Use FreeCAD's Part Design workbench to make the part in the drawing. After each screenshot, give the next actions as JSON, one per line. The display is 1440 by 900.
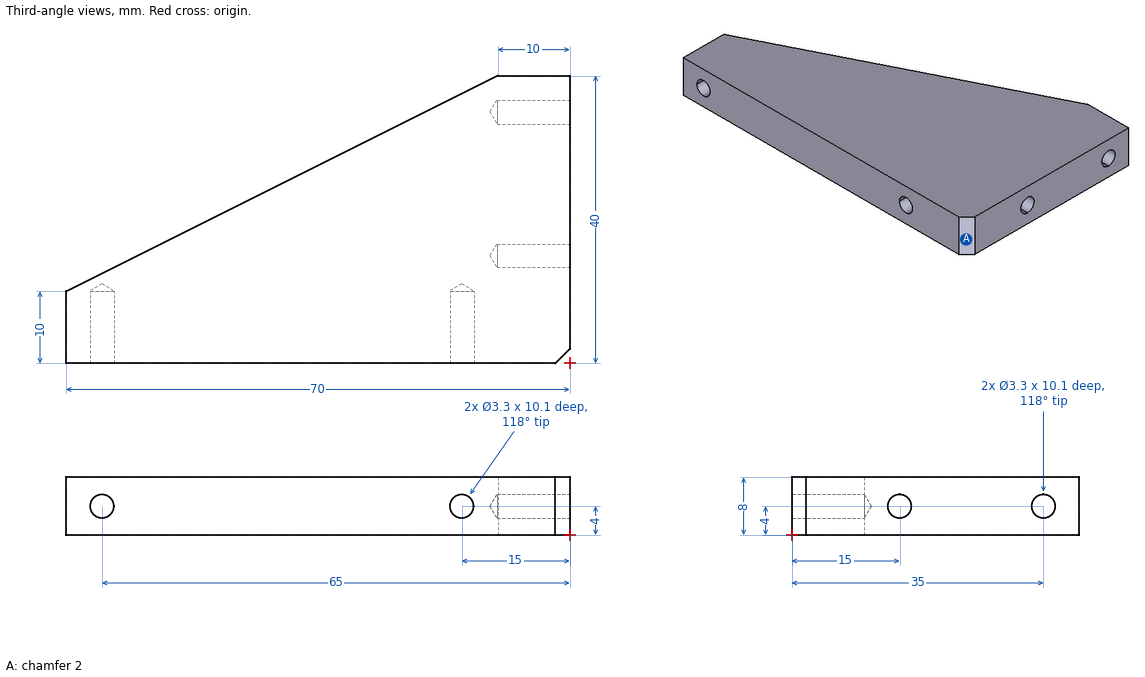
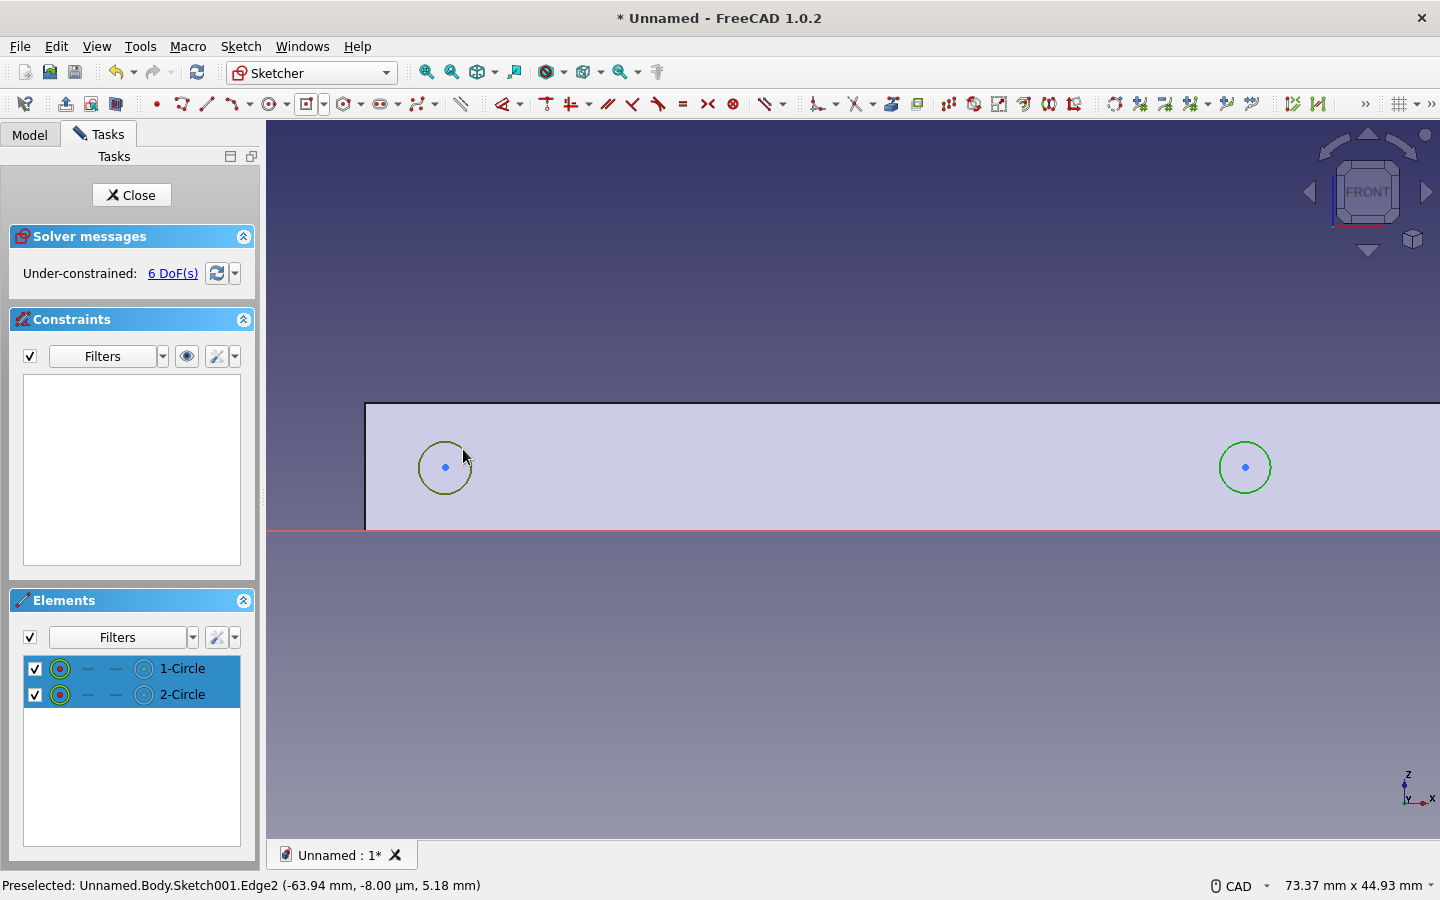
{"action": "left_click", "coordinate": [683, 104]}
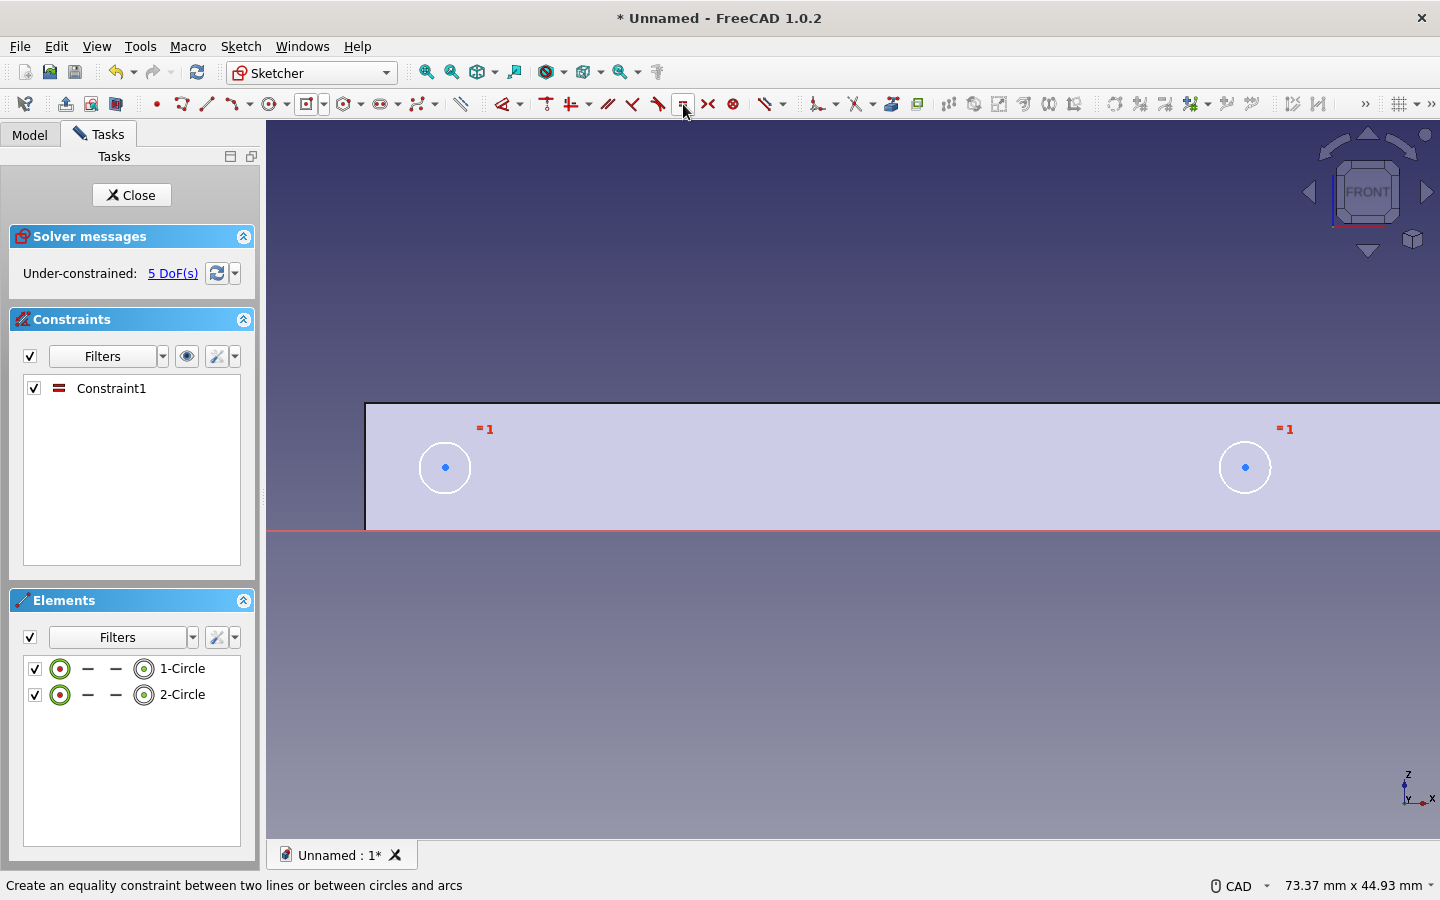
{"action": "left_click", "coordinate": [1245, 467]}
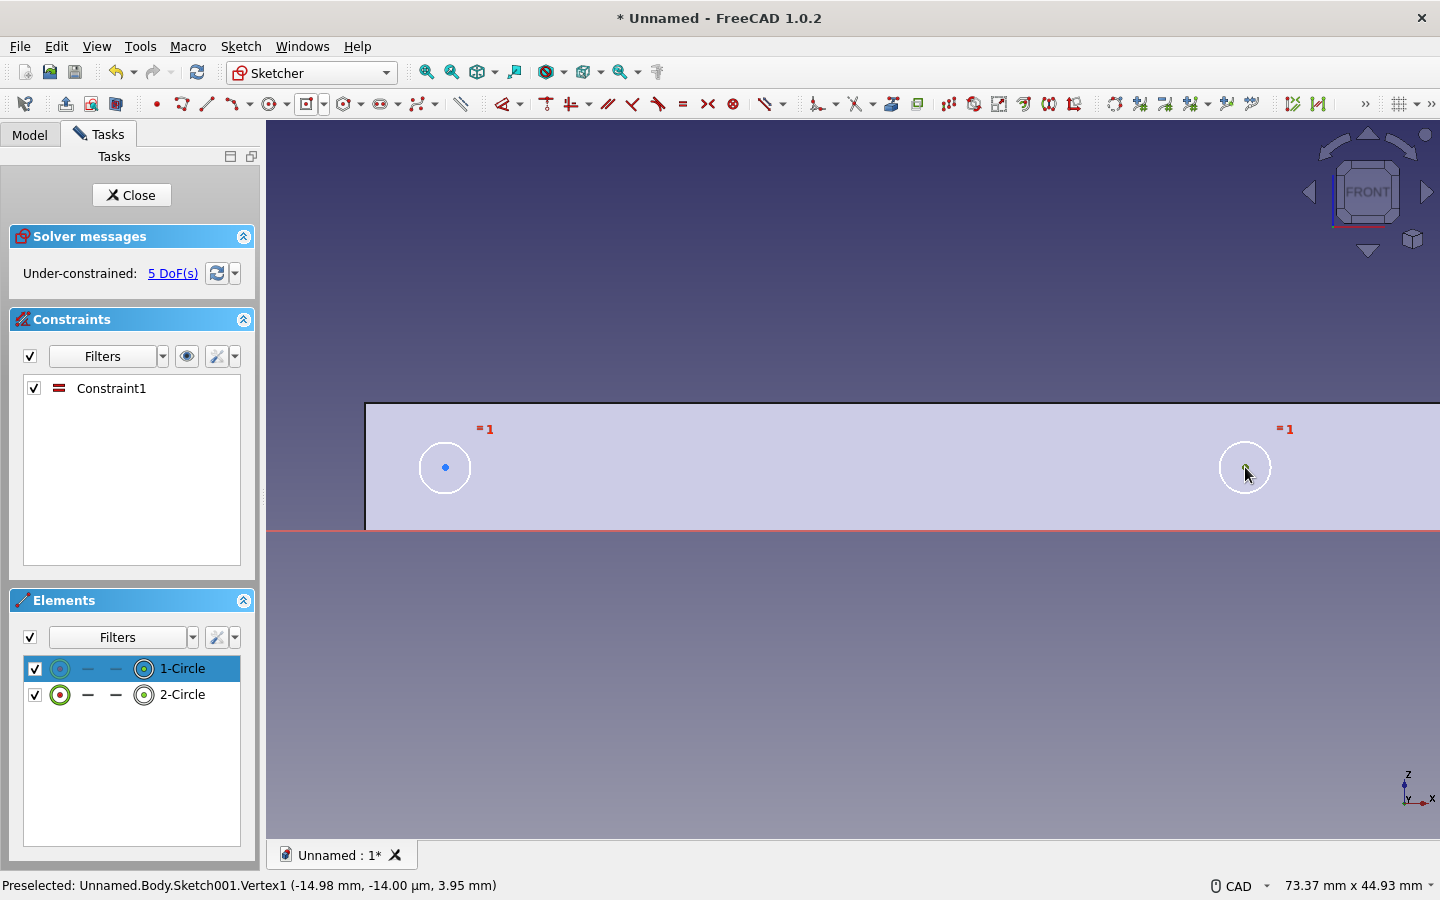
{"action": "left_click", "coordinate": [445, 468]}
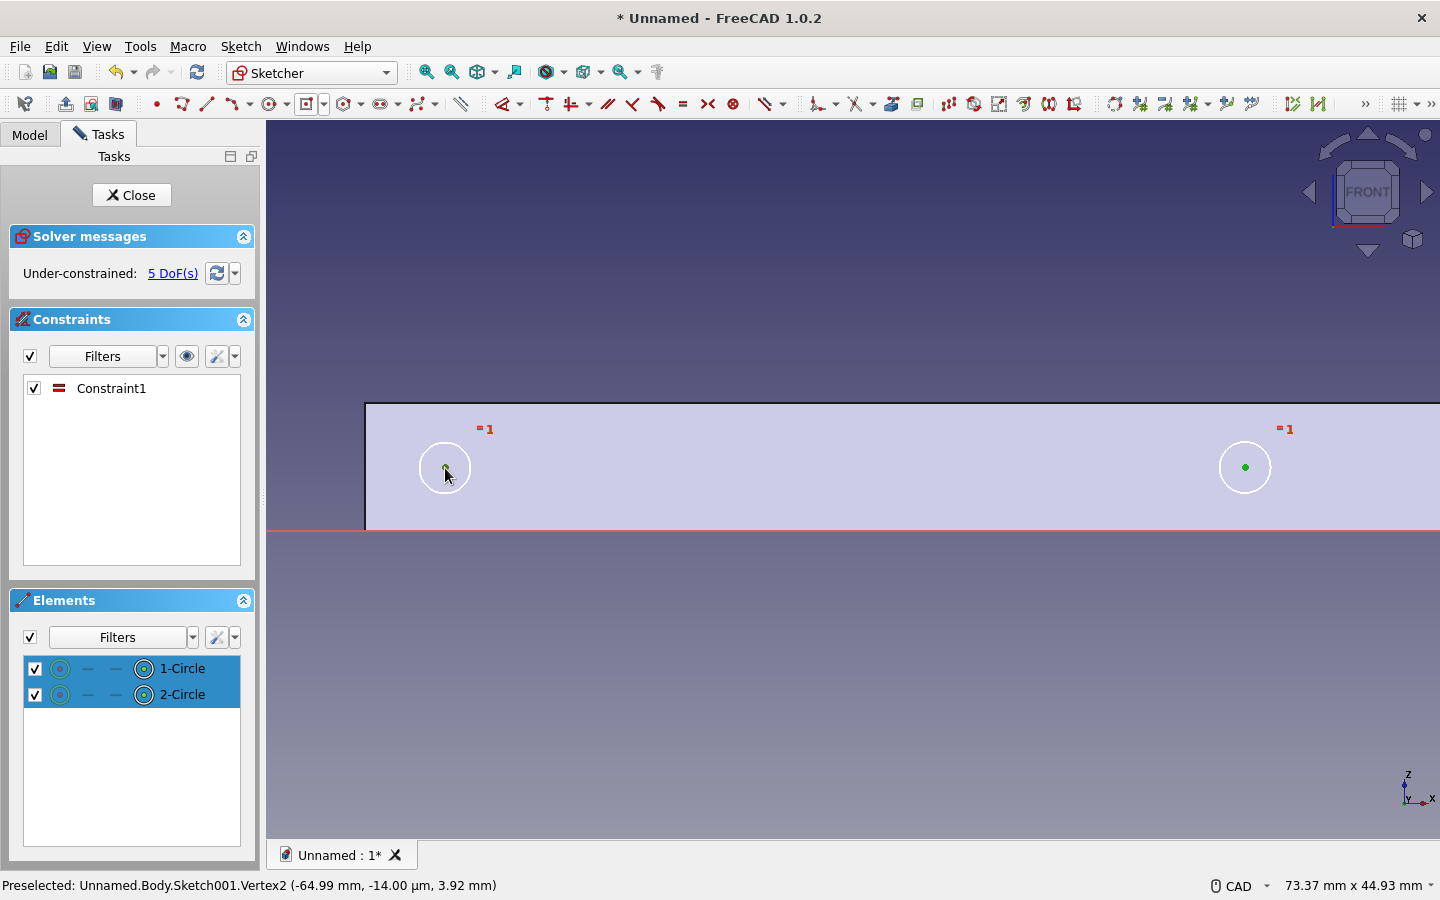
{"action": "key", "text": "h"}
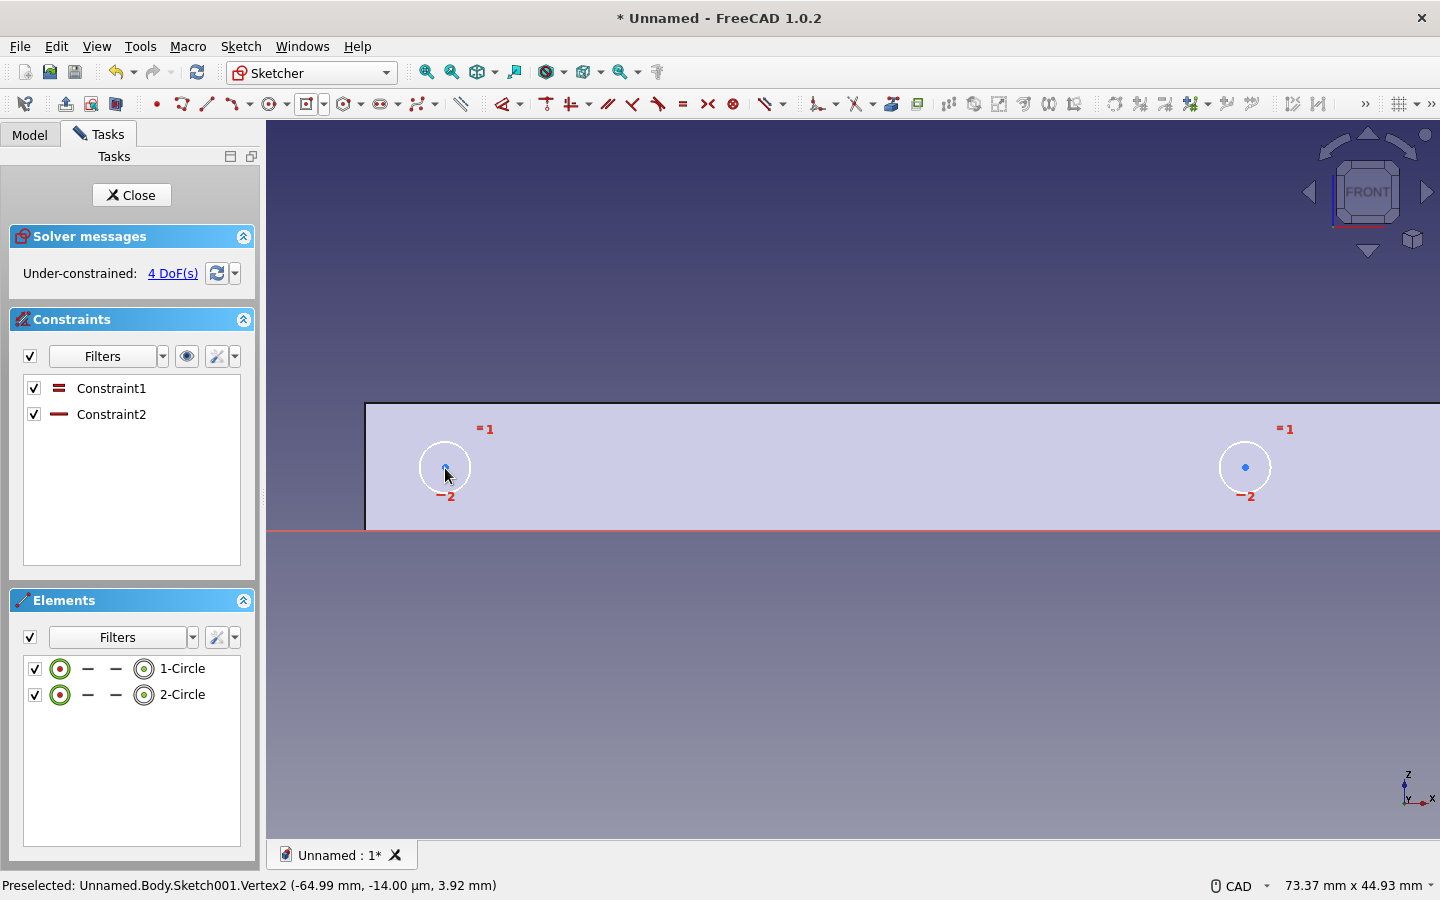
{"action": "left_click", "coordinate": [502, 104]}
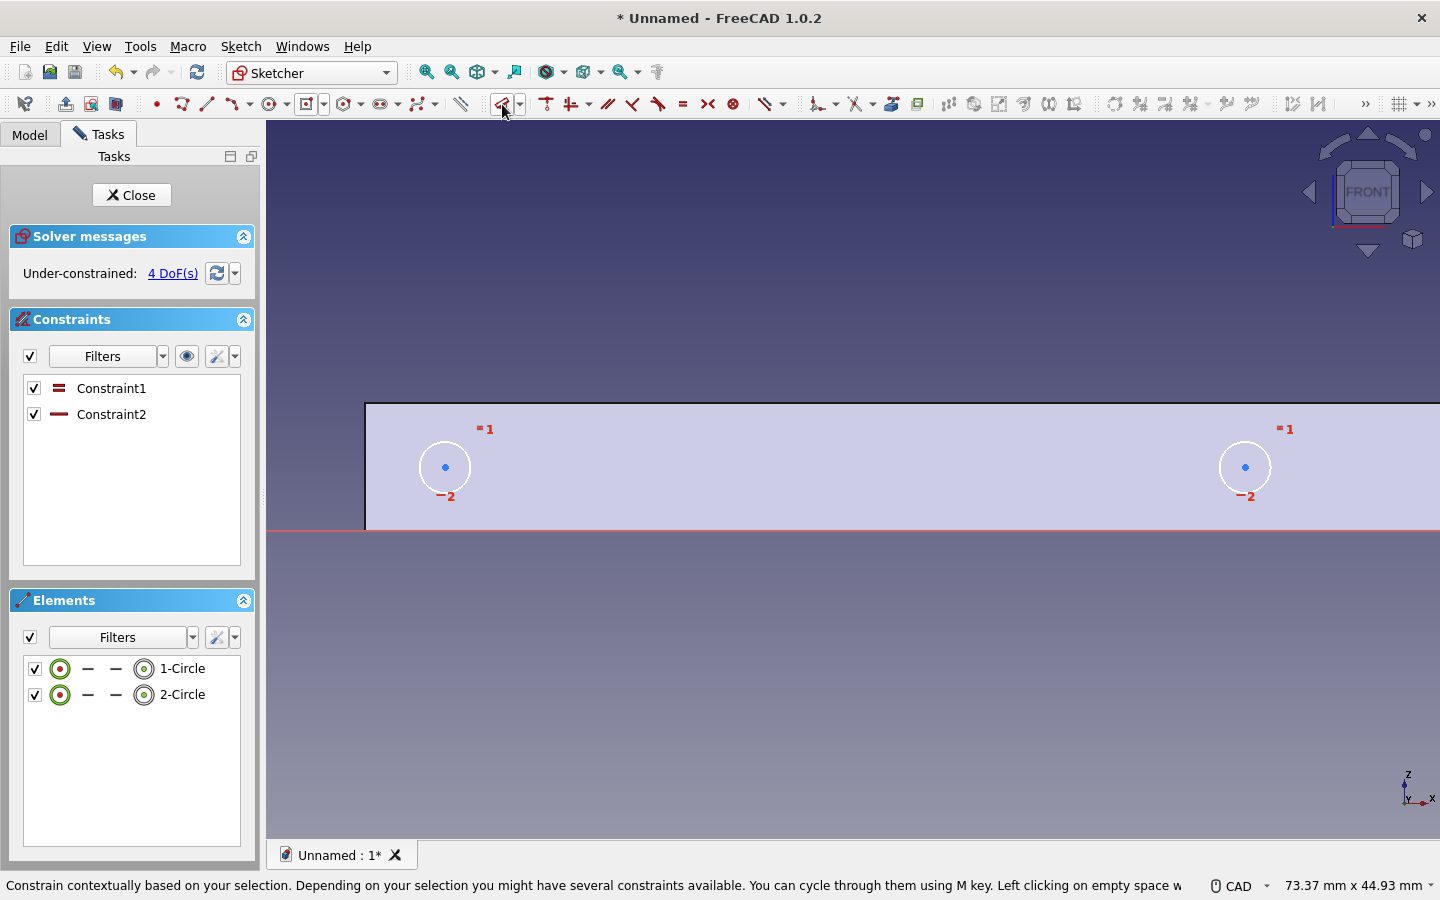
{"action": "left_click", "coordinate": [1263, 449]}
{"action": "left_click", "coordinate": [1260, 412]}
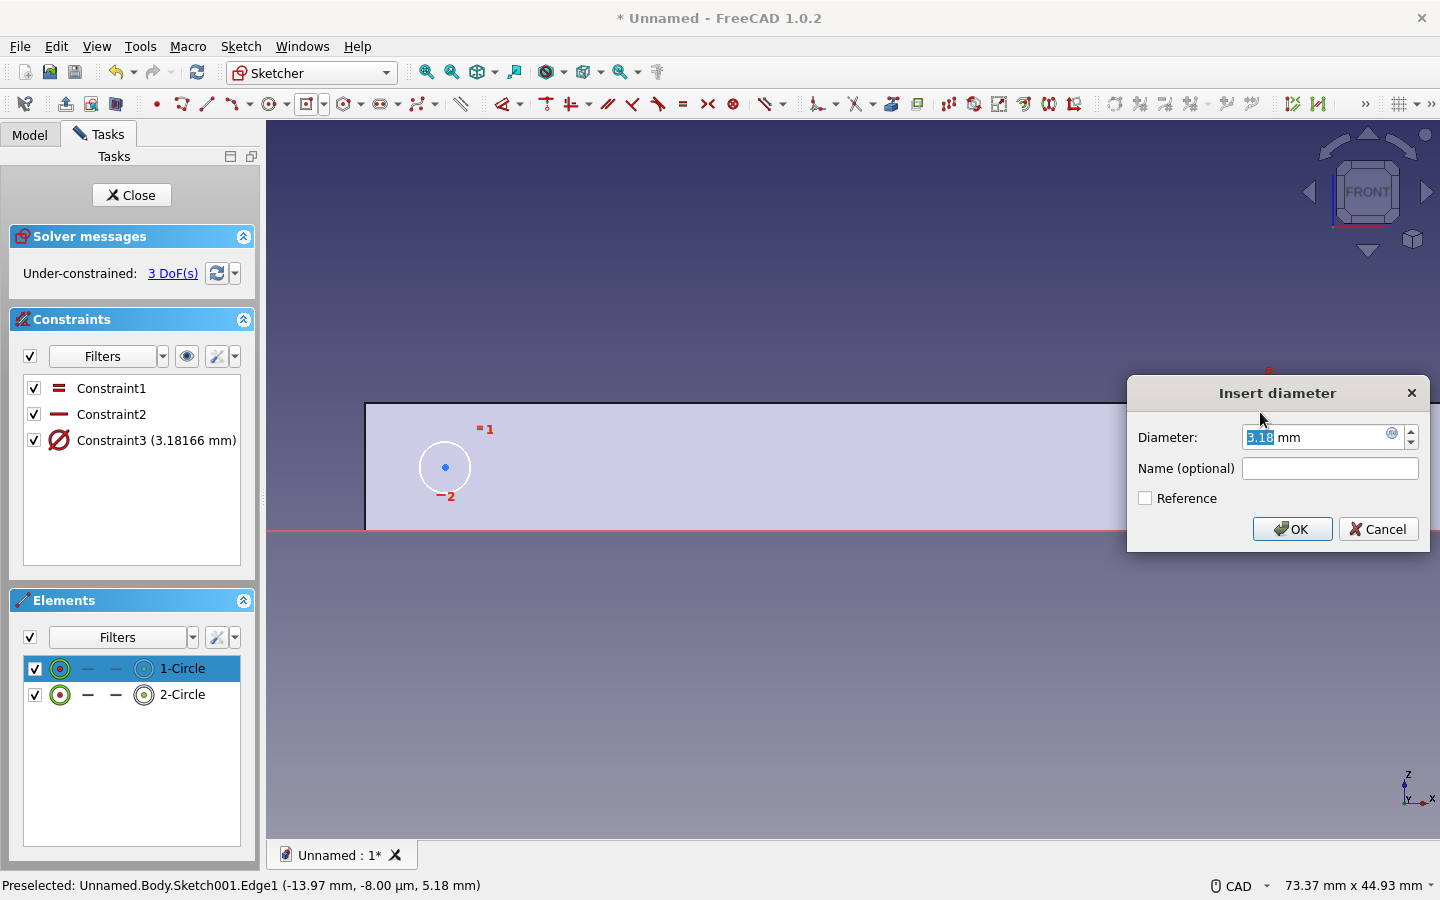
{"action": "type", "text": "3.3"}
{"action": "key", "text": "Return"}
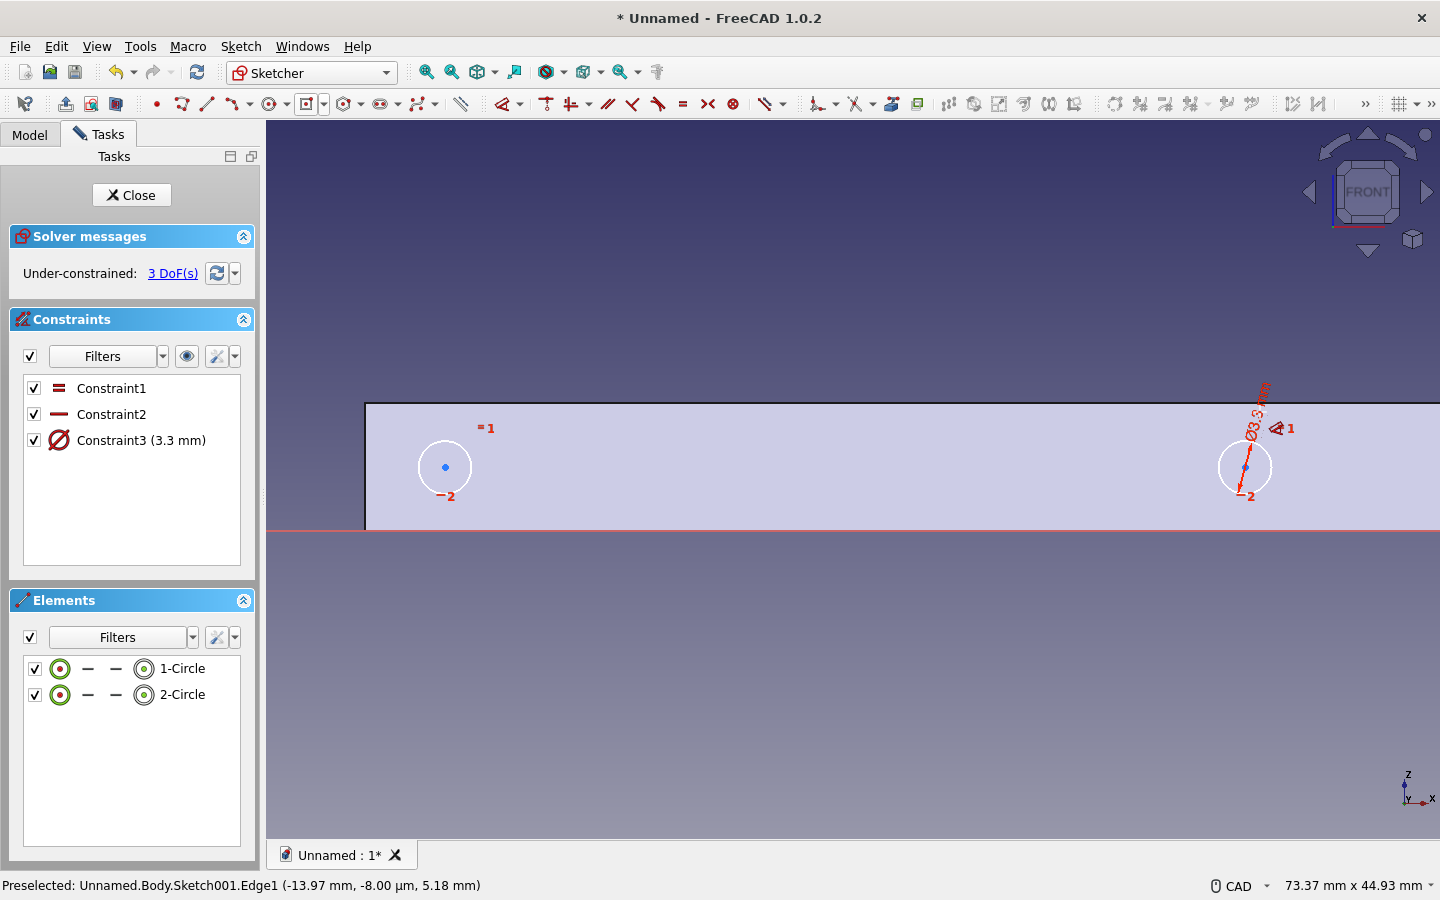
{"action": "left_click", "coordinate": [1245, 467]}
{"action": "left_click", "coordinate": [1211, 499]}